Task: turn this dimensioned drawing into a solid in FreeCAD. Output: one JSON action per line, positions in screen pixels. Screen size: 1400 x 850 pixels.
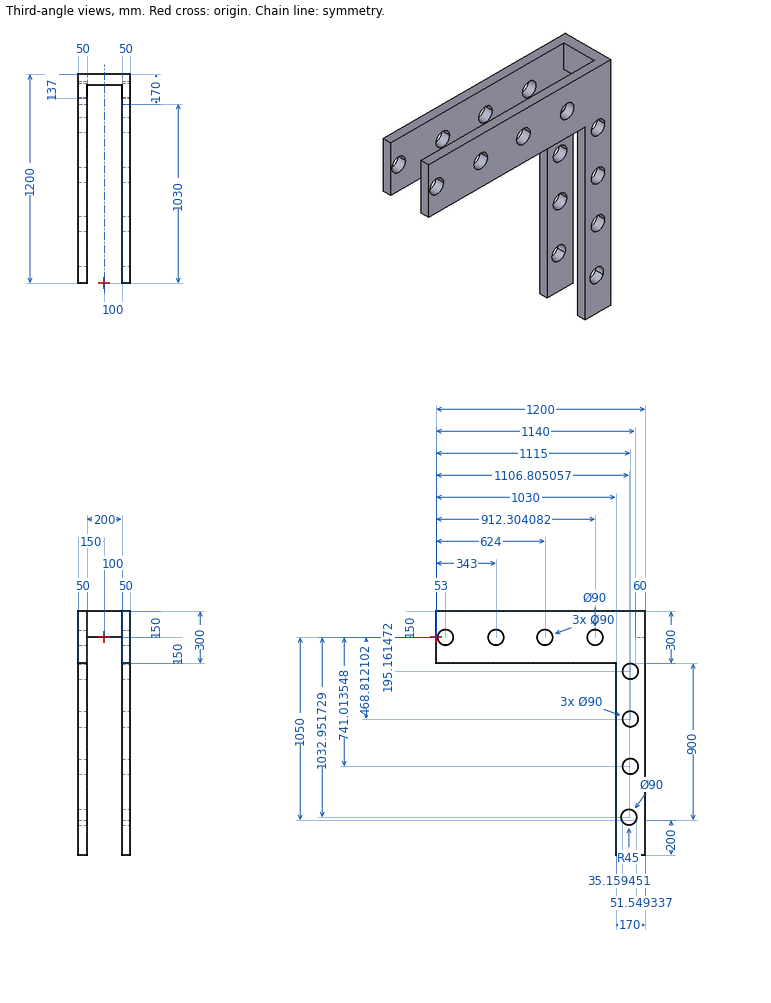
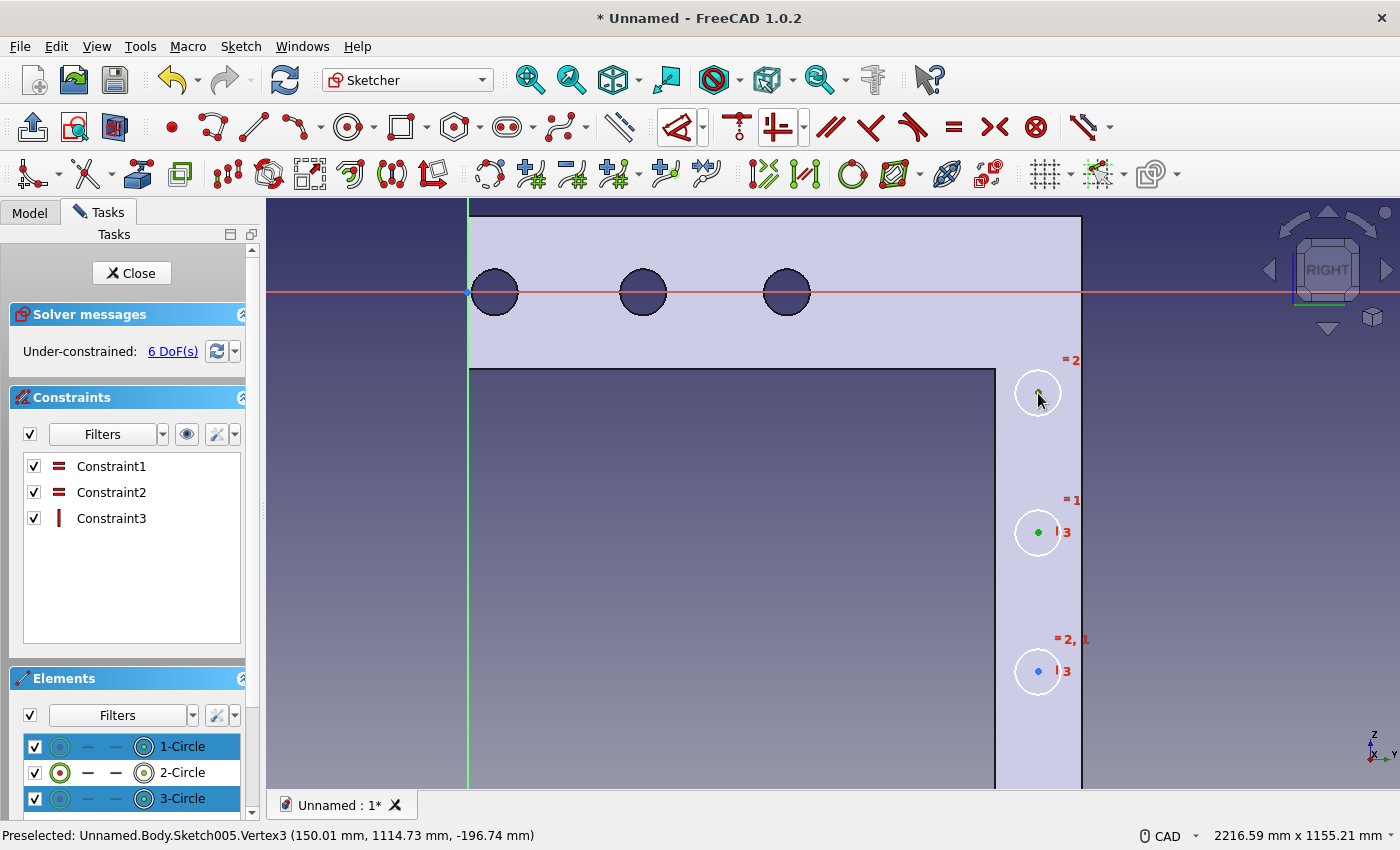
{"action": "left_click", "coordinate": [804, 128]}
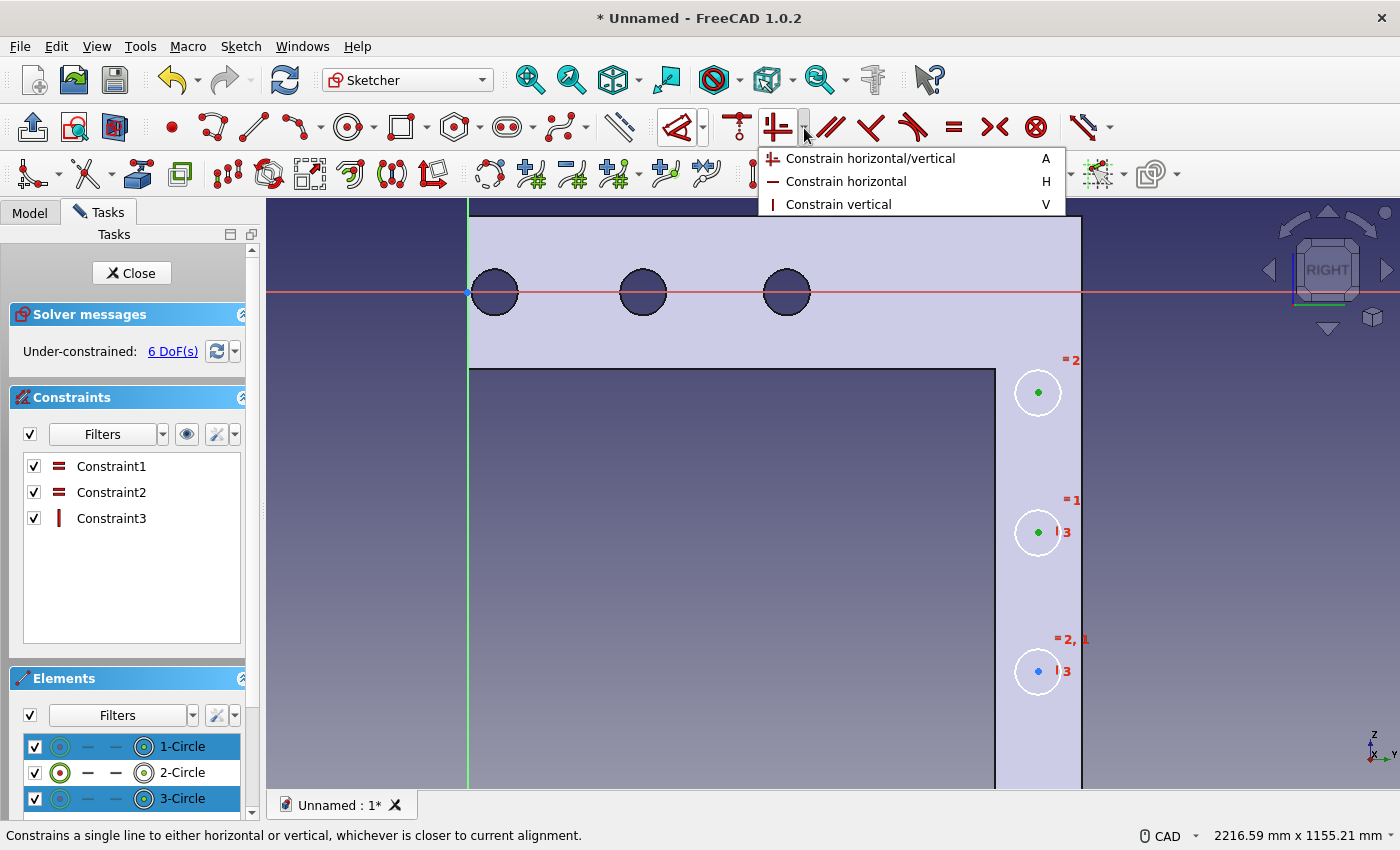
{"action": "left_click", "coordinate": [912, 204]}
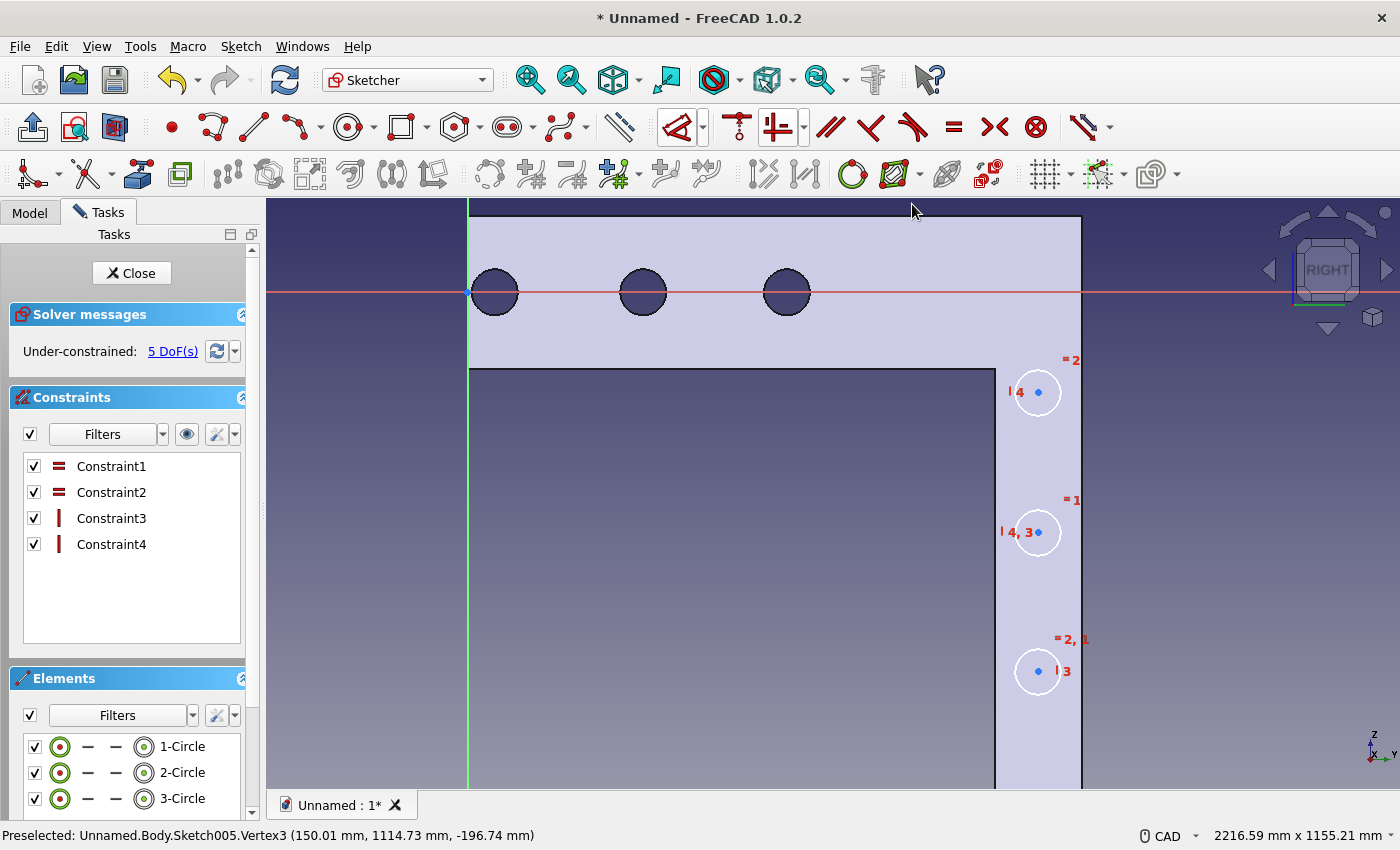
{"action": "left_click", "coordinate": [1054, 517]}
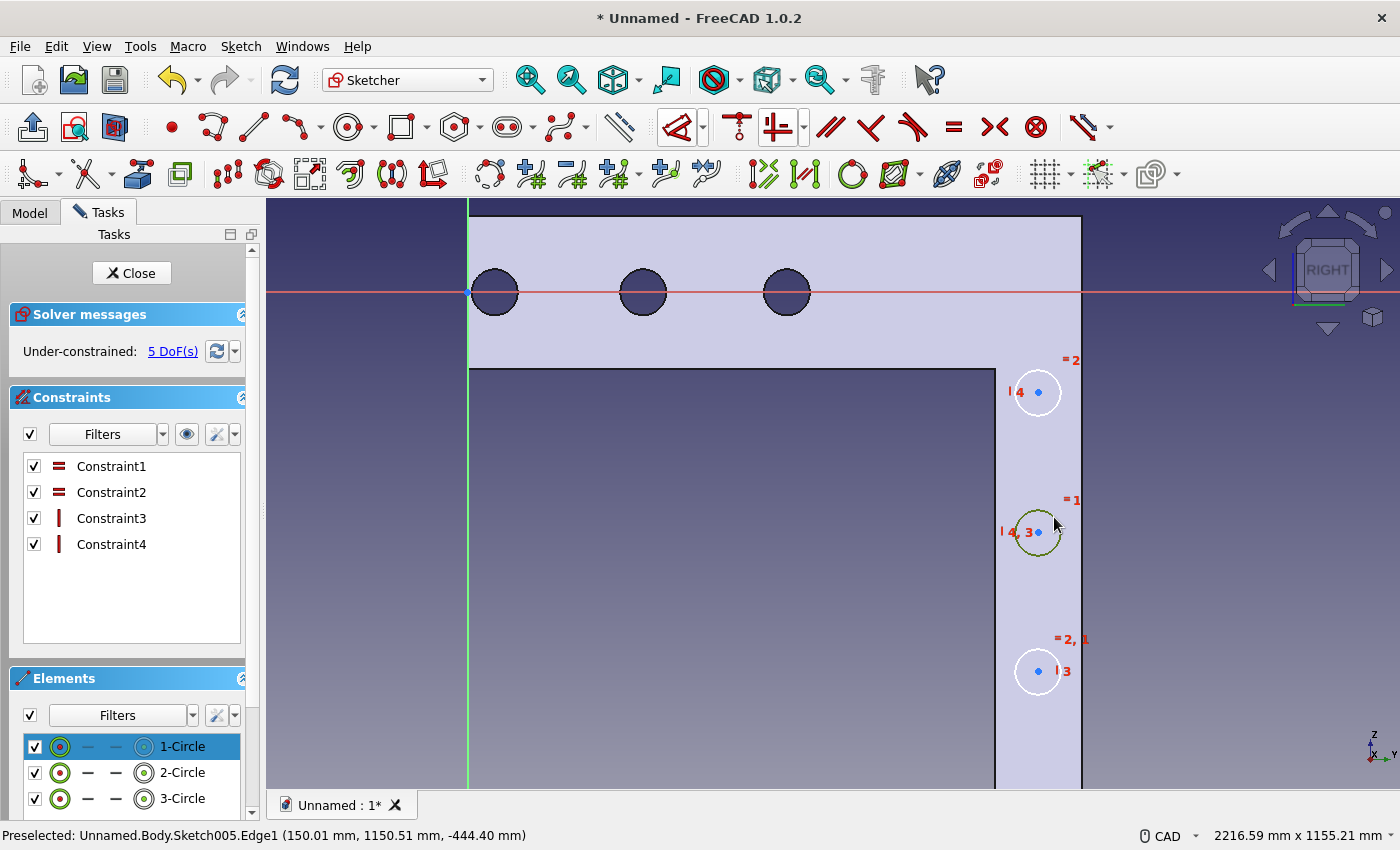
{"action": "key", "text": "k o"}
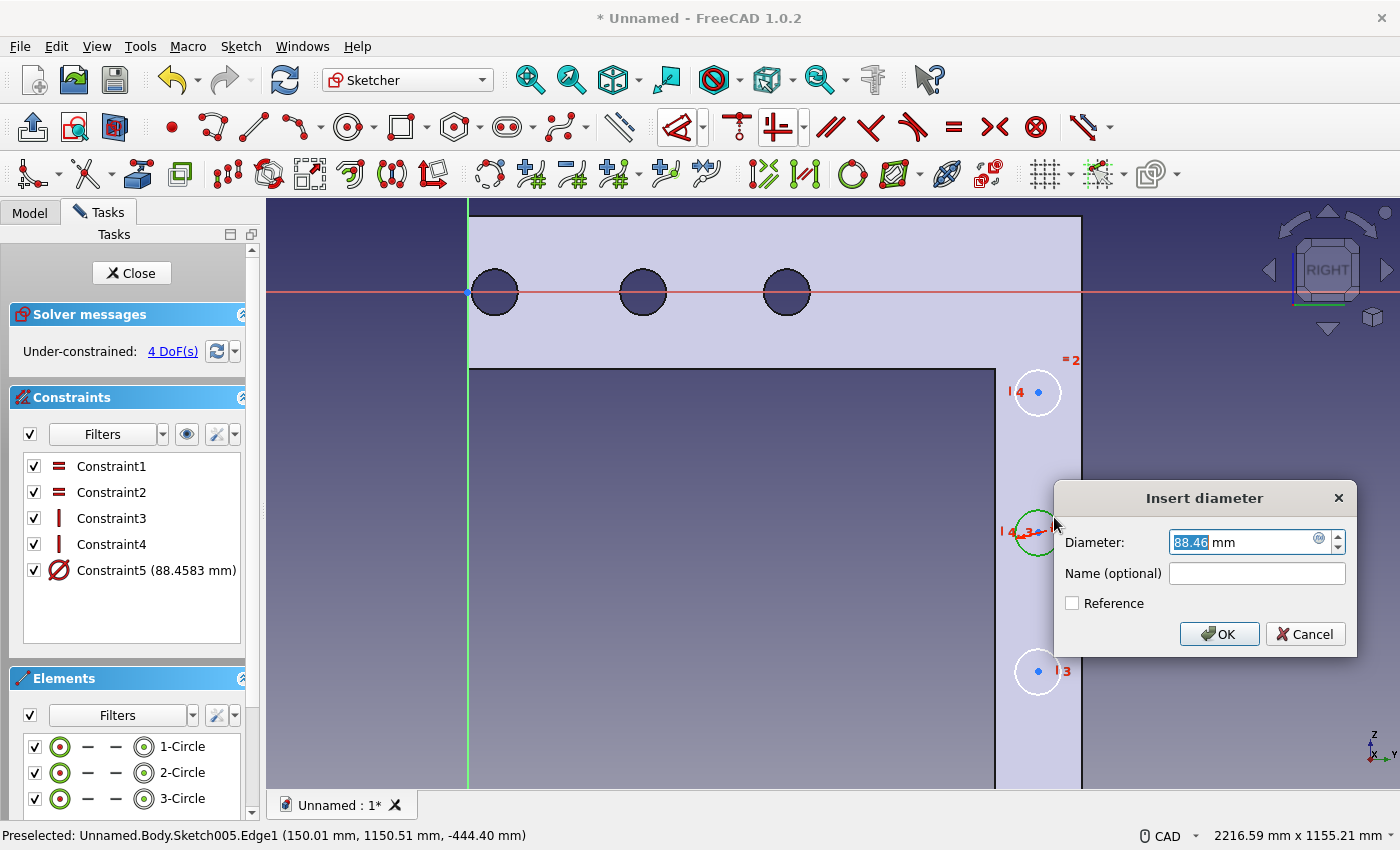
{"action": "type", "text": "90"}
{"action": "key", "text": "Return"}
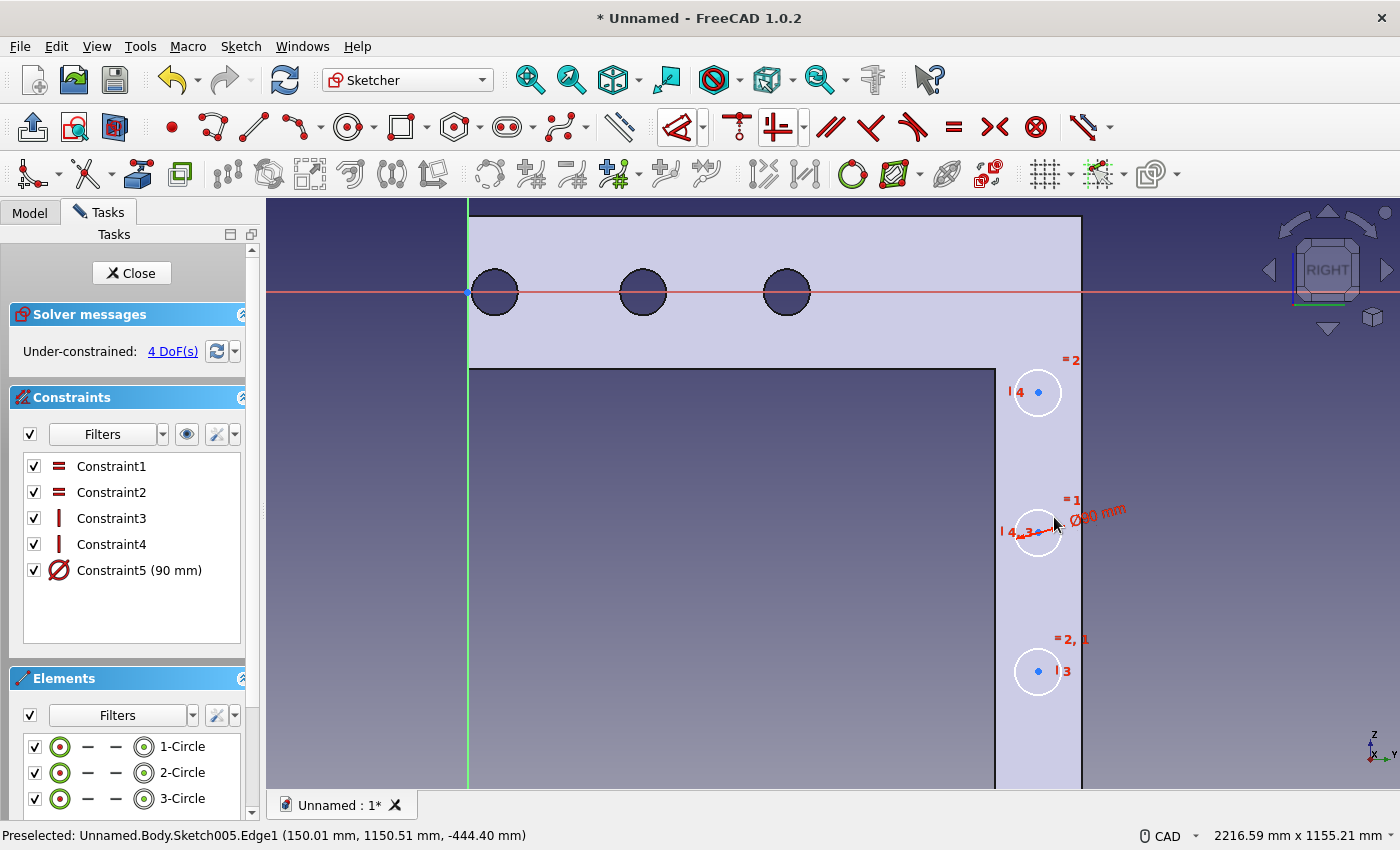
{"action": "left_click", "coordinate": [1038, 533]}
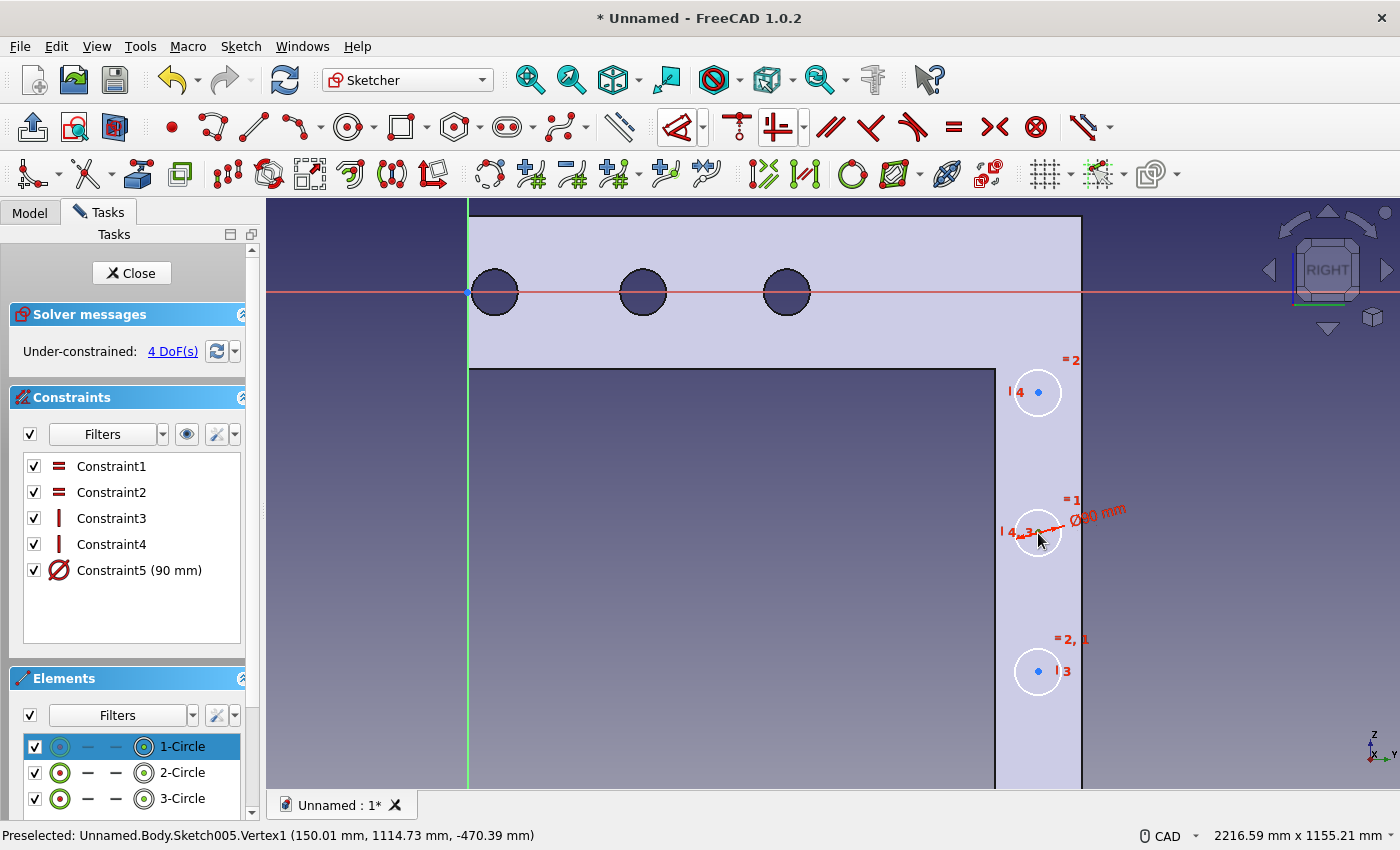
{"action": "left_click", "coordinate": [702, 128]}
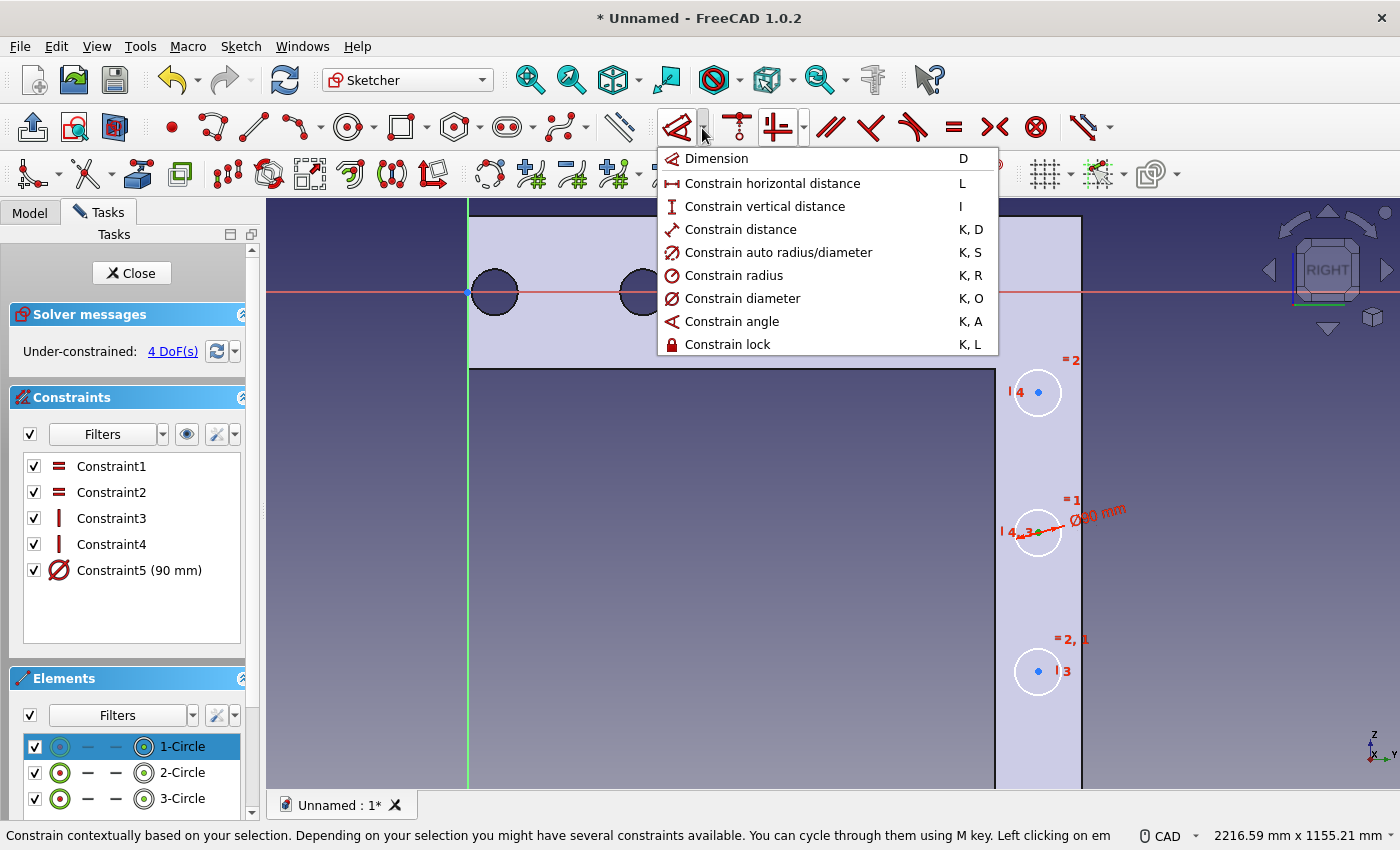
{"action": "left_click", "coordinate": [828, 184]}